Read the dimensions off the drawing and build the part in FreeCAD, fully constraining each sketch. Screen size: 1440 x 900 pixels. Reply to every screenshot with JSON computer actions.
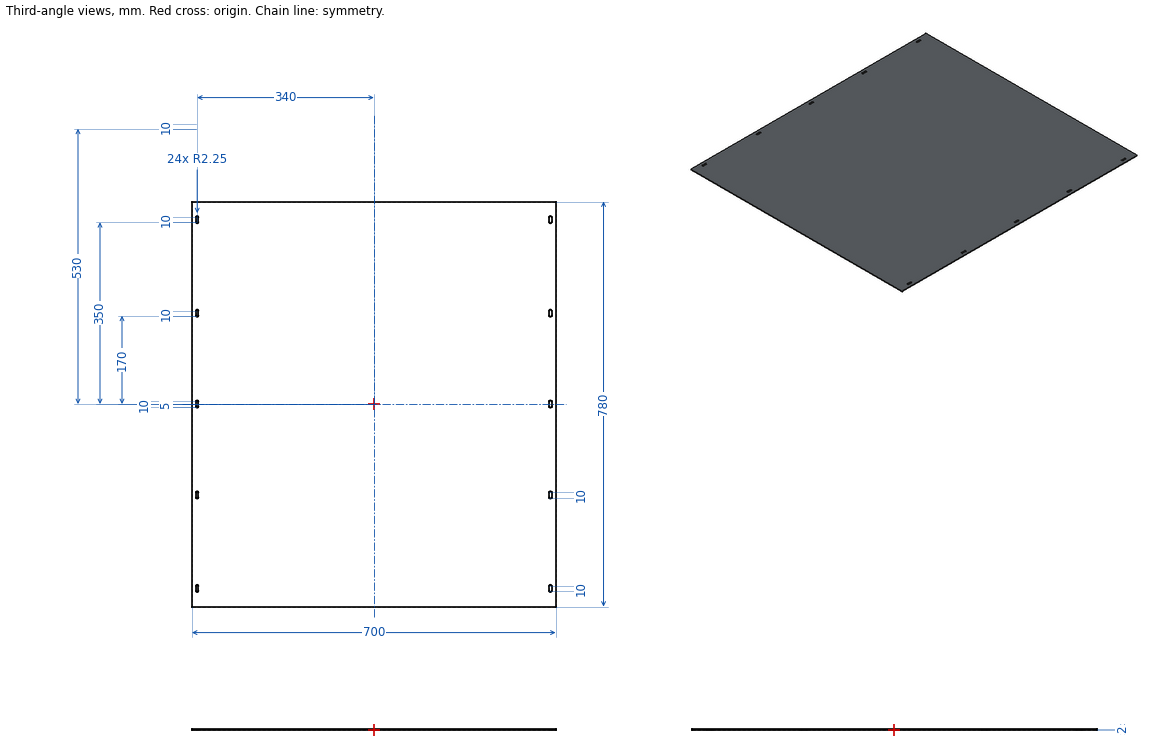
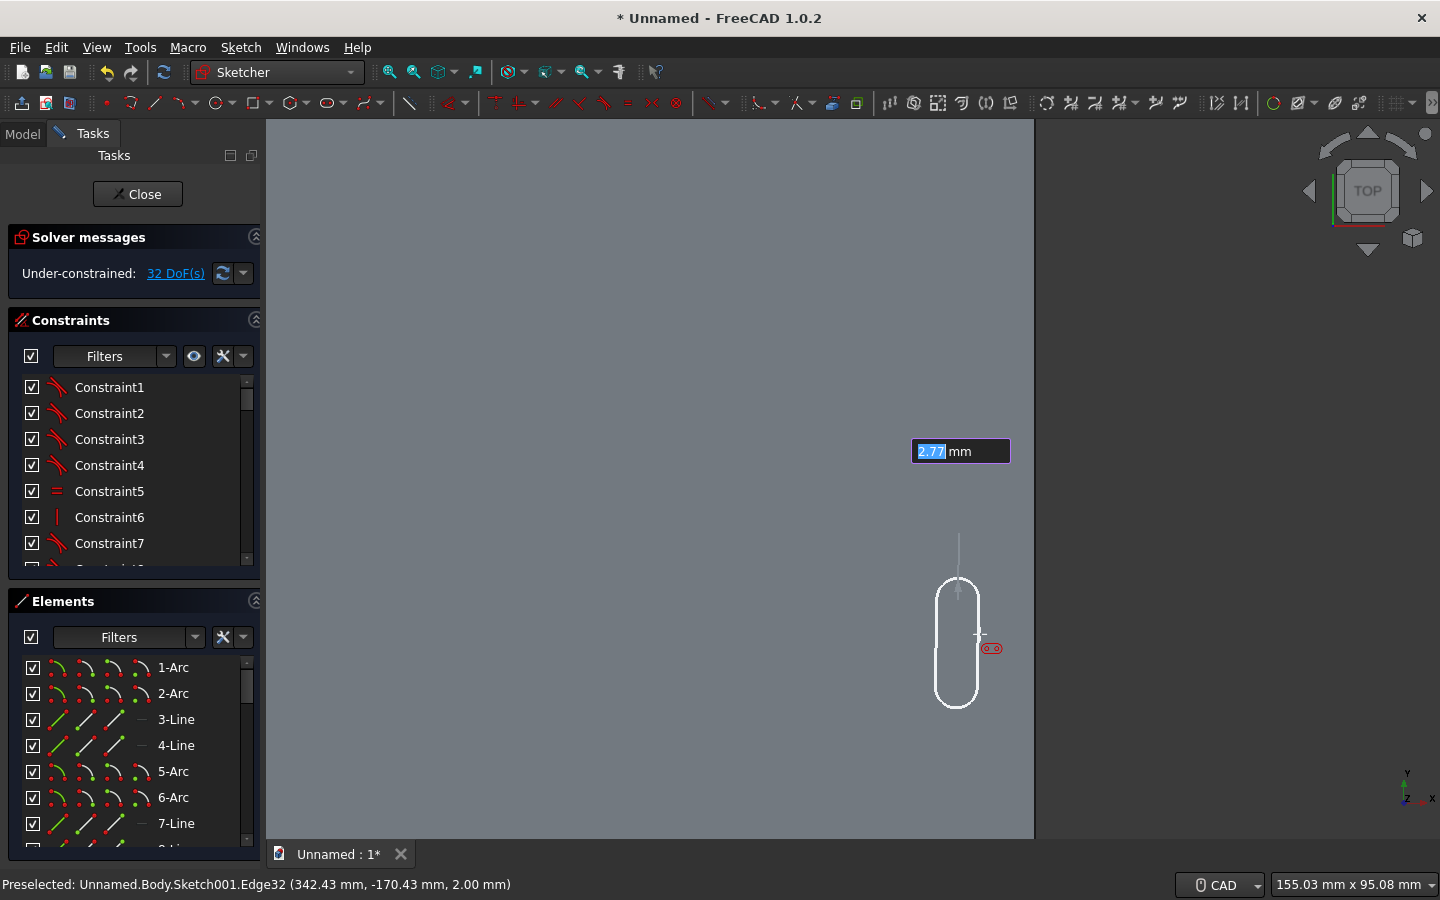
{"action": "left_click", "coordinate": [976, 633]}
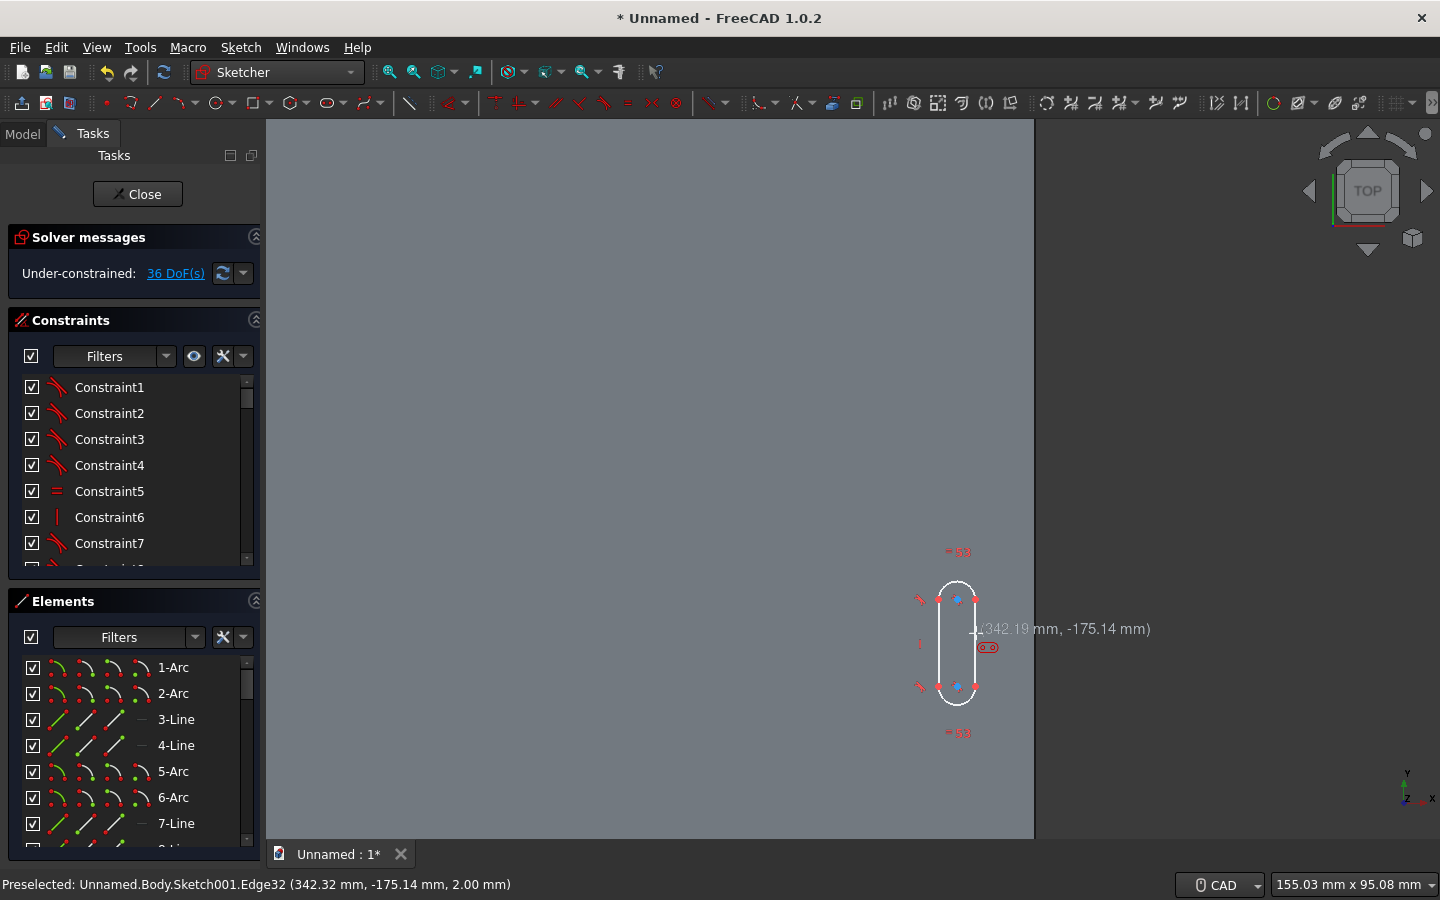
{"action": "scroll", "coordinate": [977, 628], "scroll_direction": "down", "scroll_amount": 13}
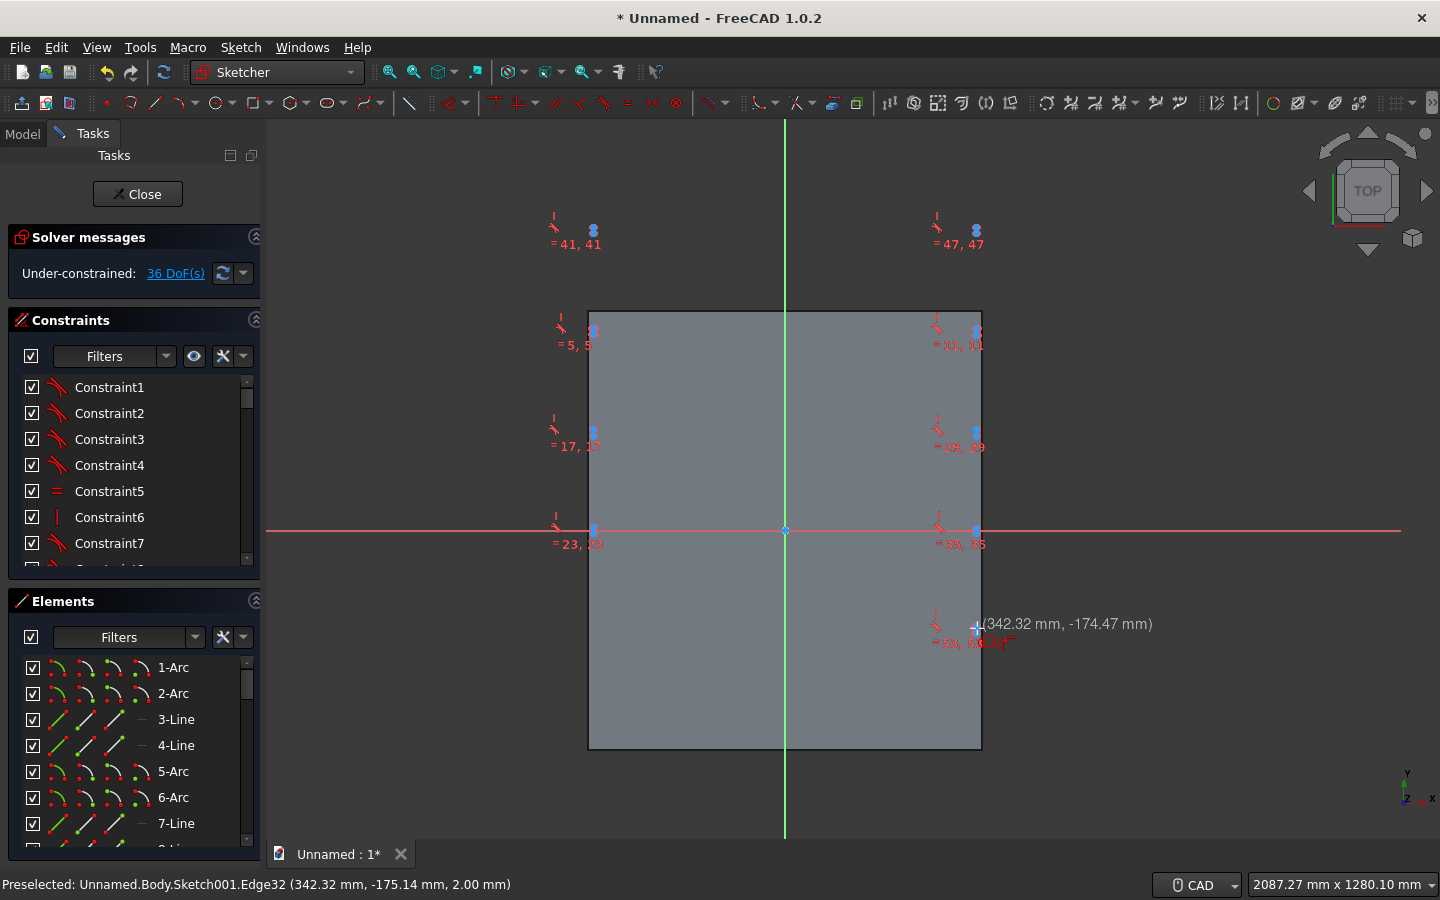
{"action": "scroll", "coordinate": [594, 632], "scroll_direction": "up", "scroll_amount": 15}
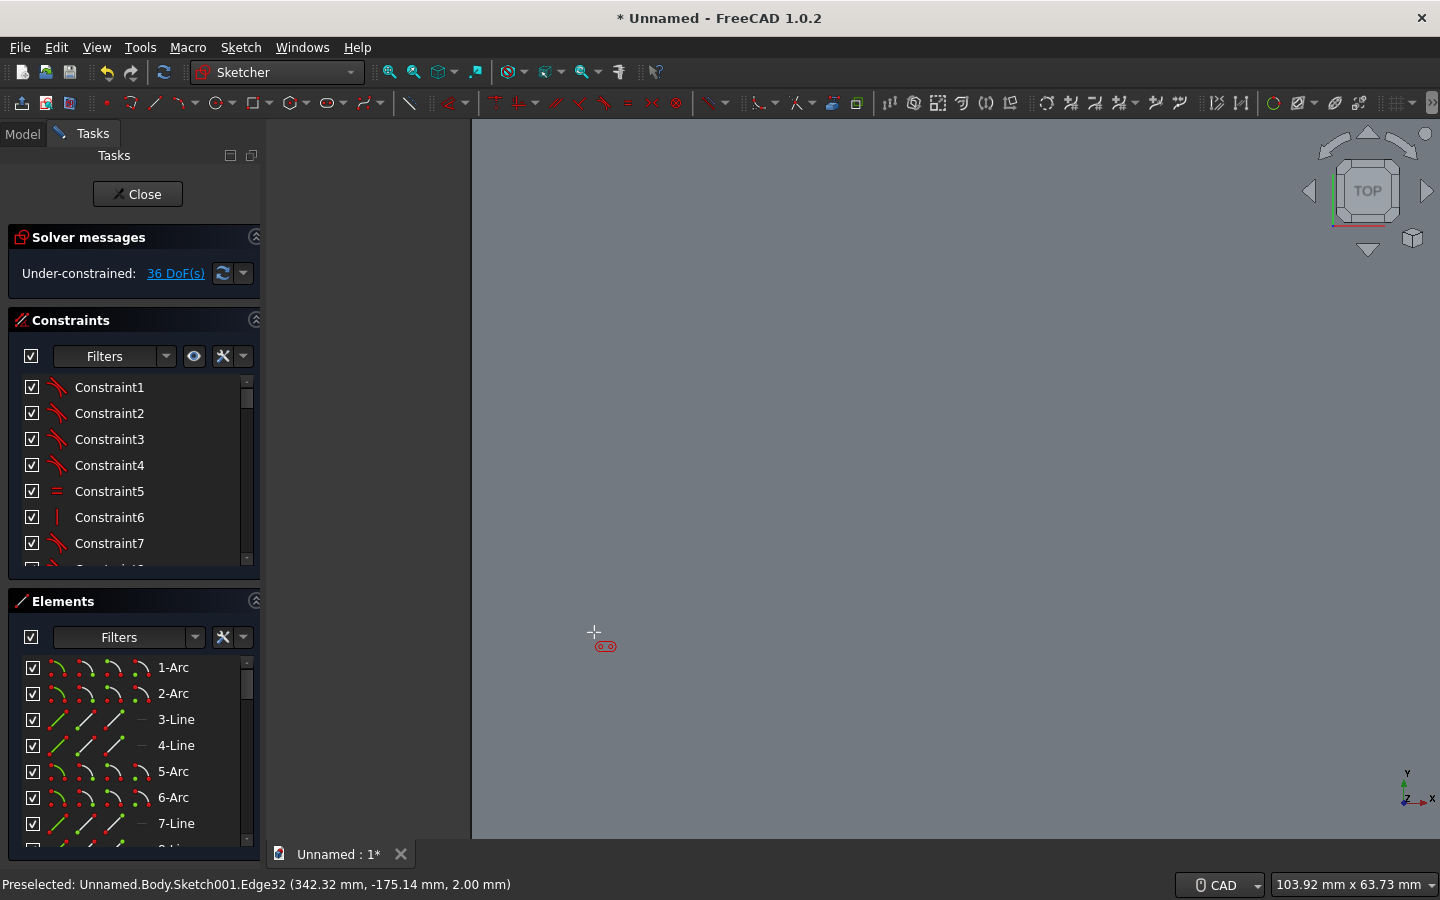
{"action": "scroll", "coordinate": [594, 632], "scroll_direction": "down", "scroll_amount": 15}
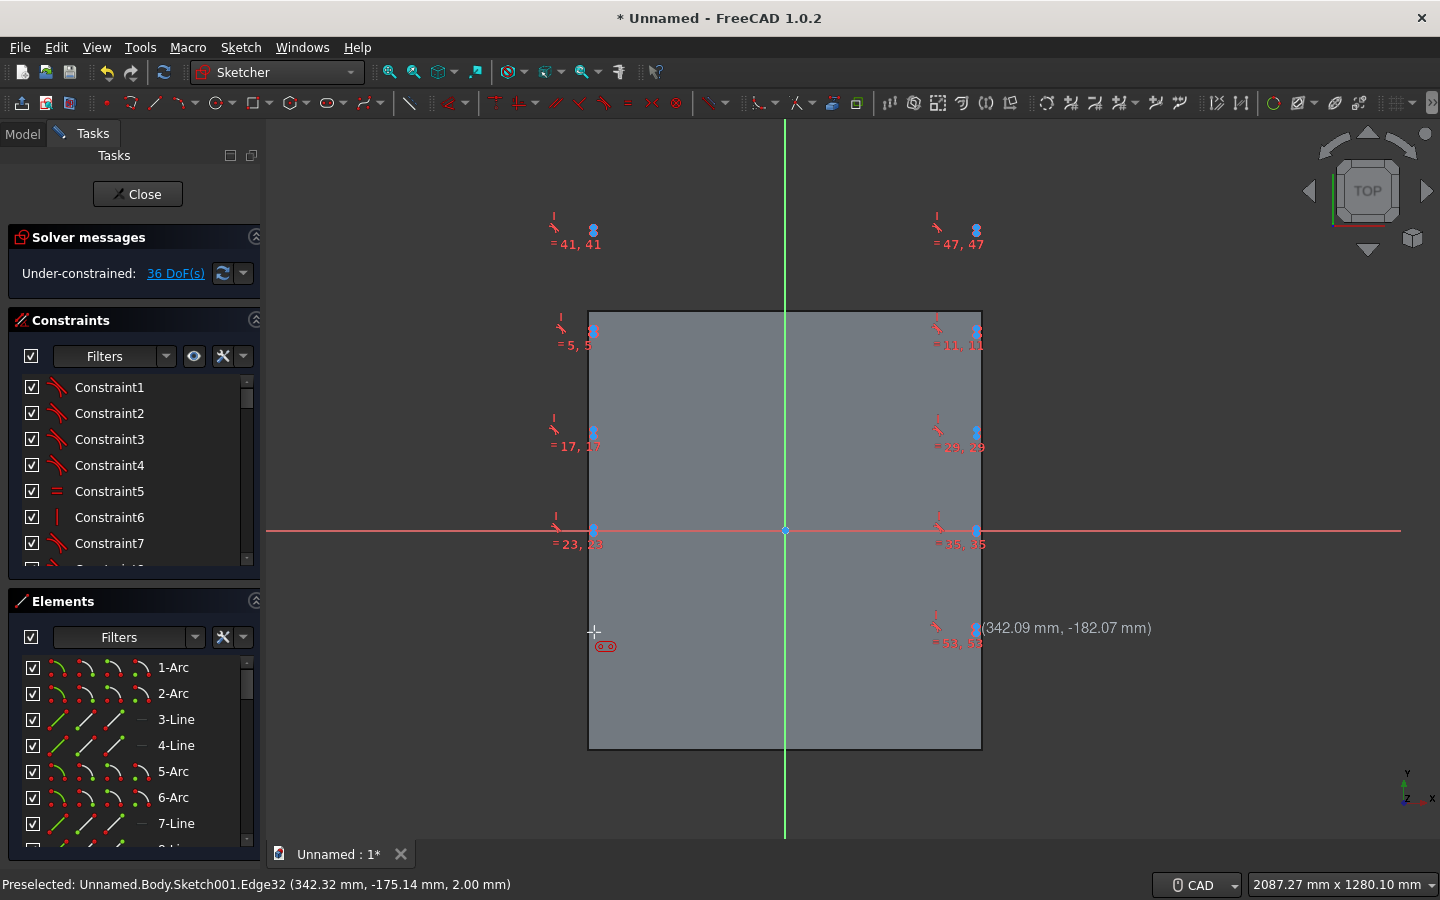
{"action": "left_click", "coordinate": [594, 632]}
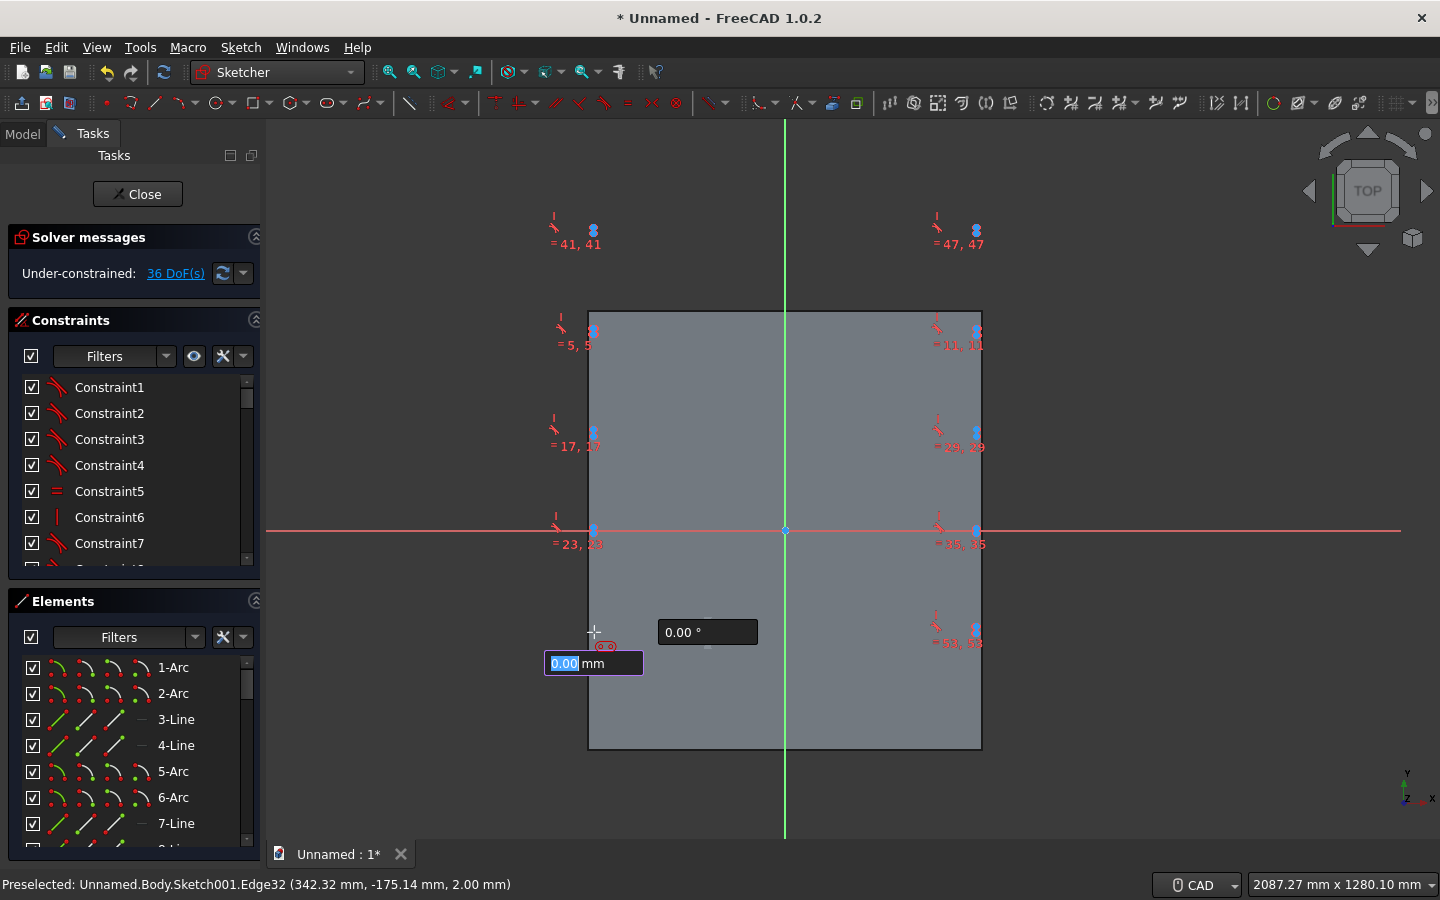
{"action": "scroll", "coordinate": [594, 626], "scroll_direction": "up", "scroll_amount": 6}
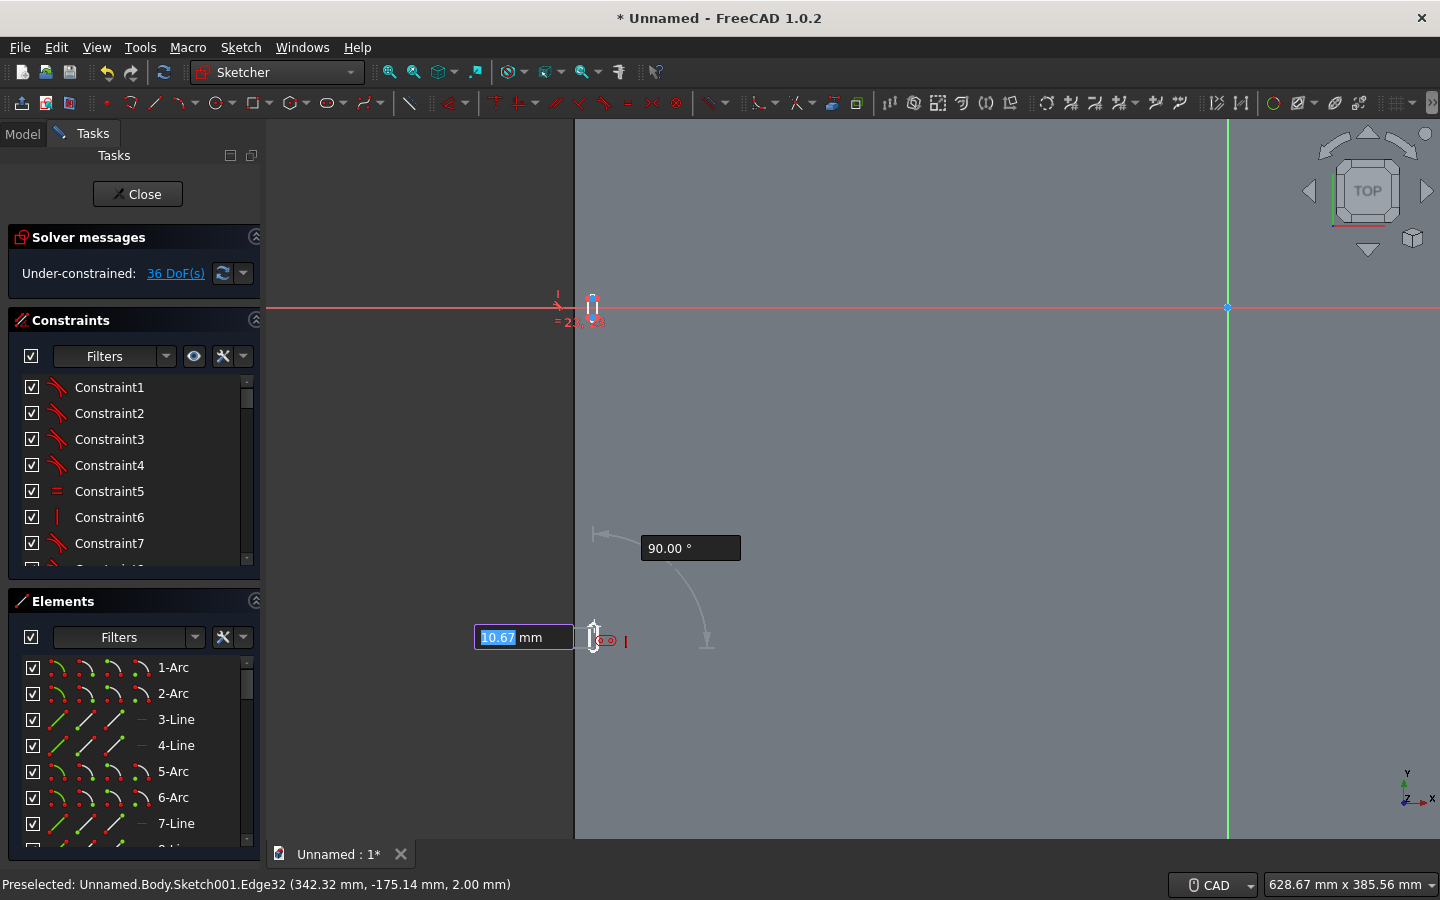
{"action": "left_click", "coordinate": [593, 625]}